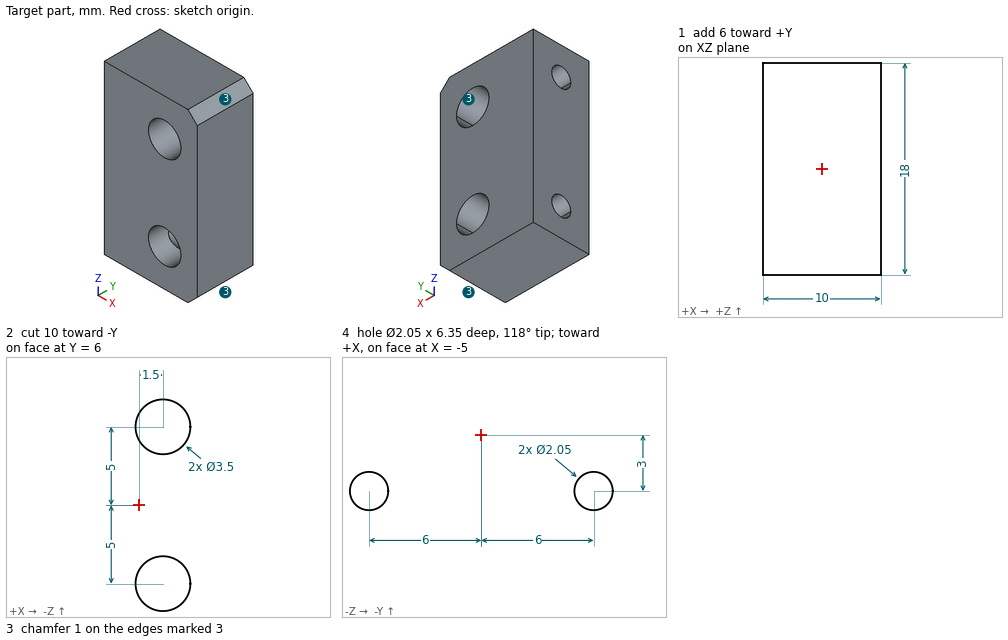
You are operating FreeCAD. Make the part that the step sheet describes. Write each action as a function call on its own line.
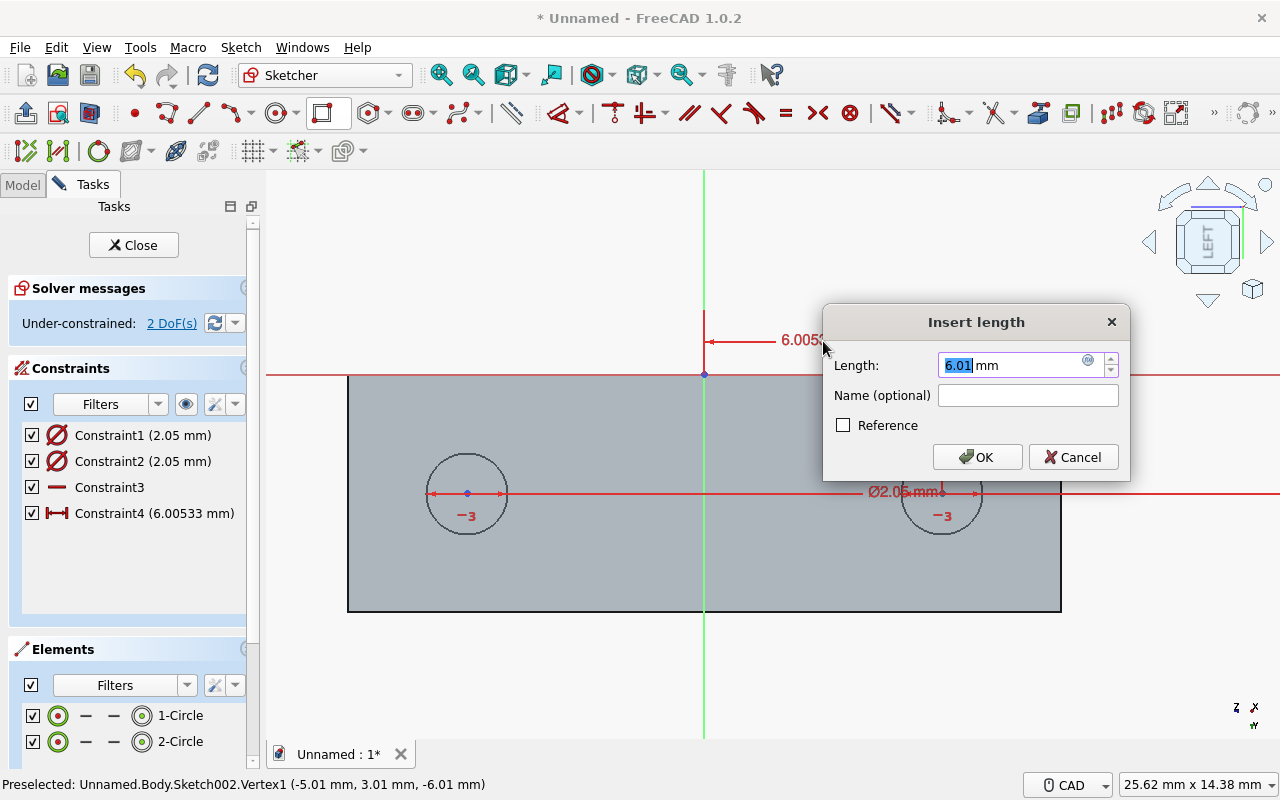
text(6)
key(Return)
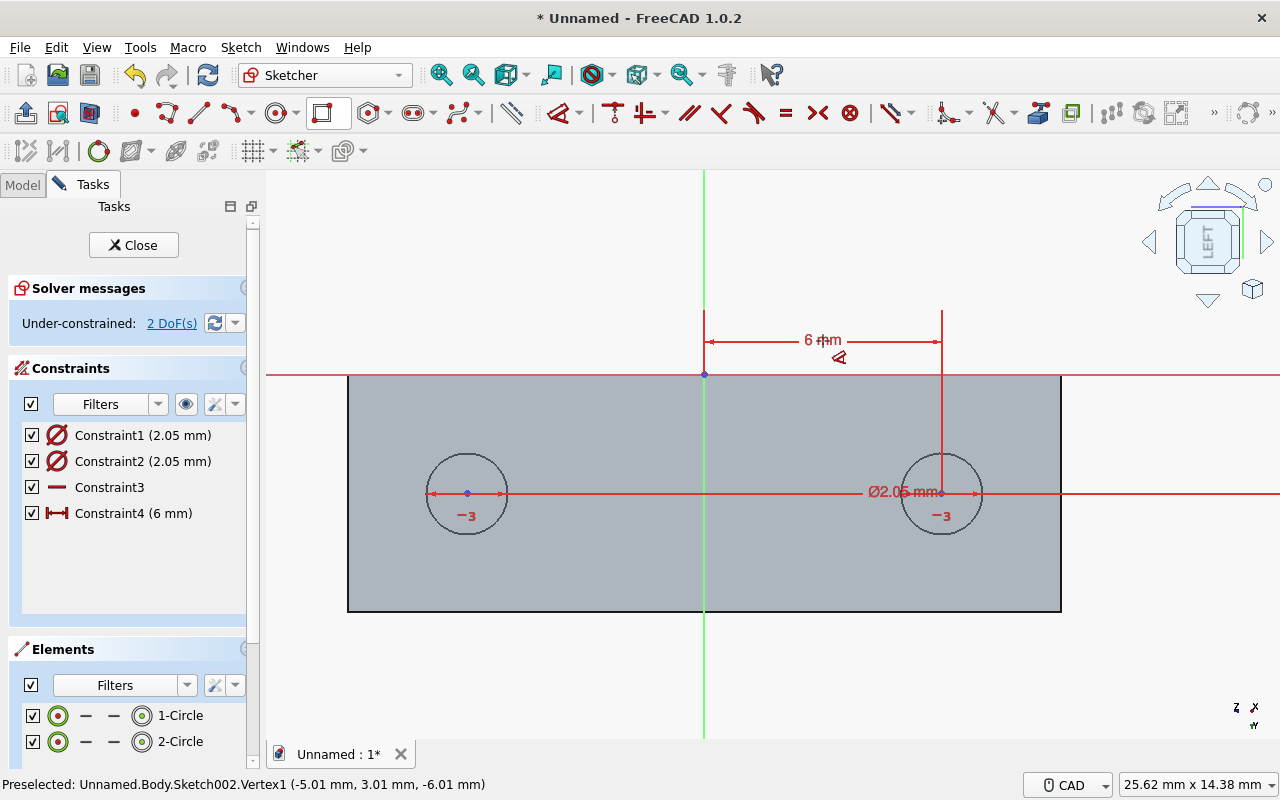
click(942, 494)
click(976, 434)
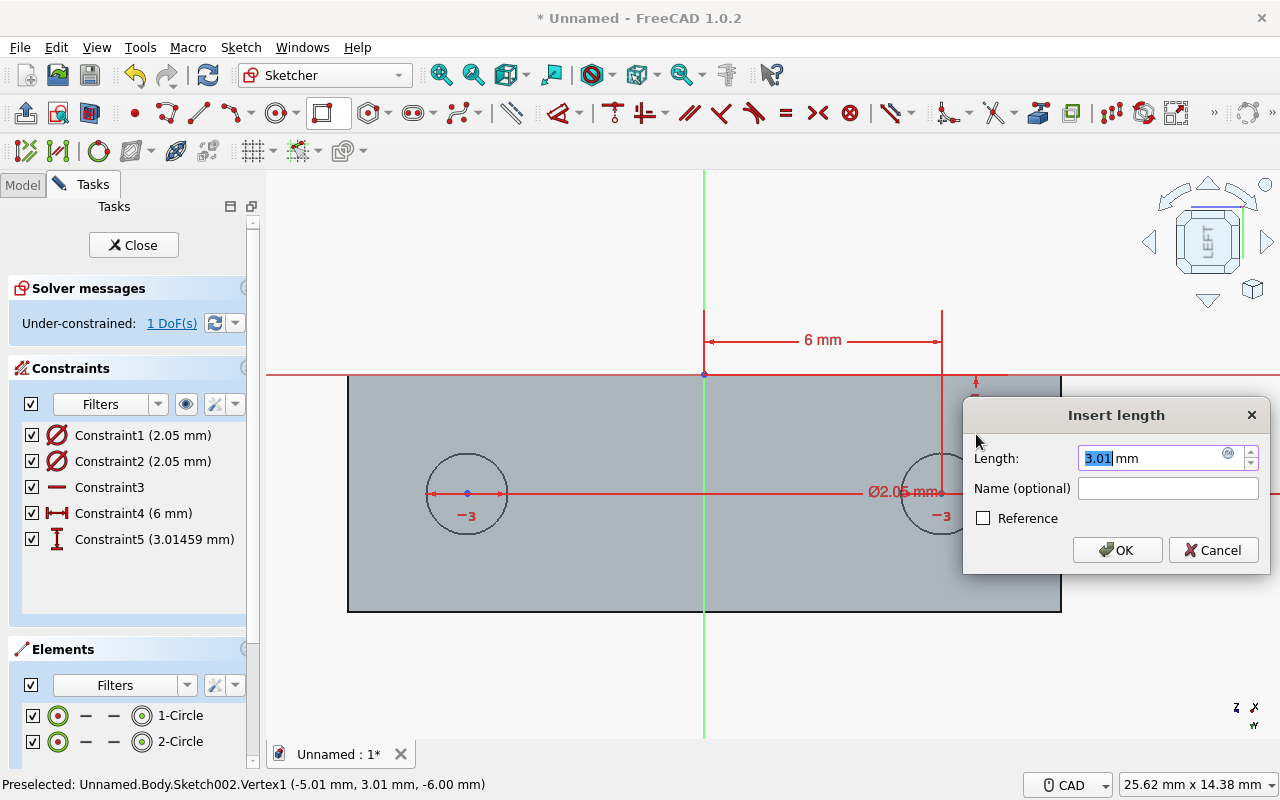
text(3)
key(Return)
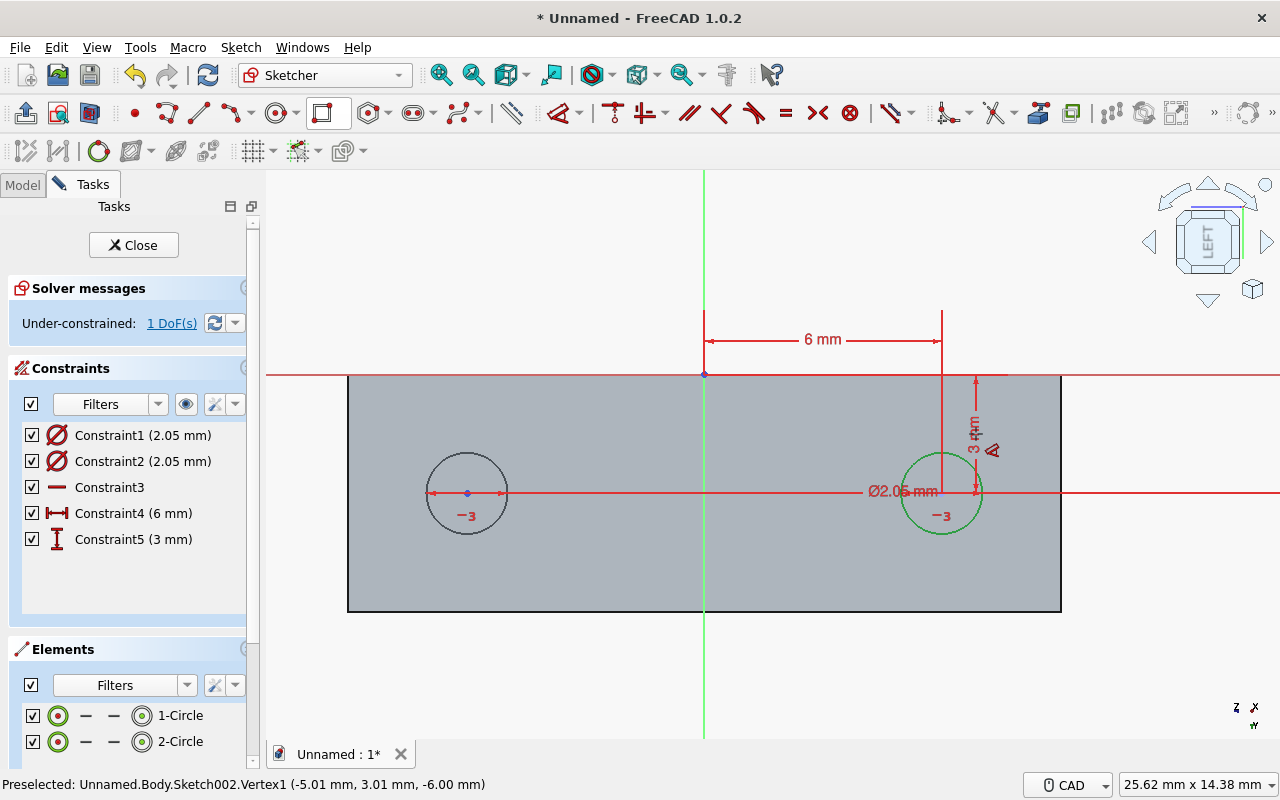
click(467, 493)
click(586, 341)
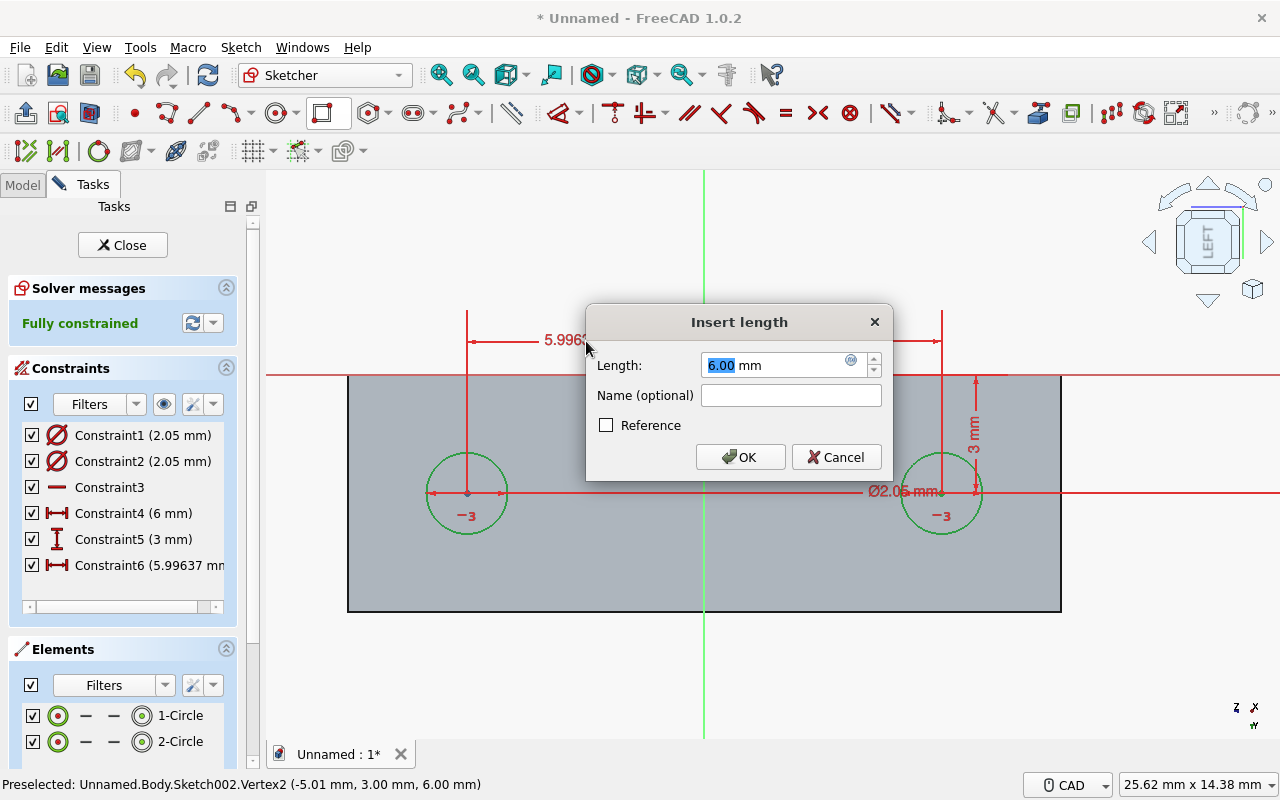
text(6)
key(Return)
key(Escape)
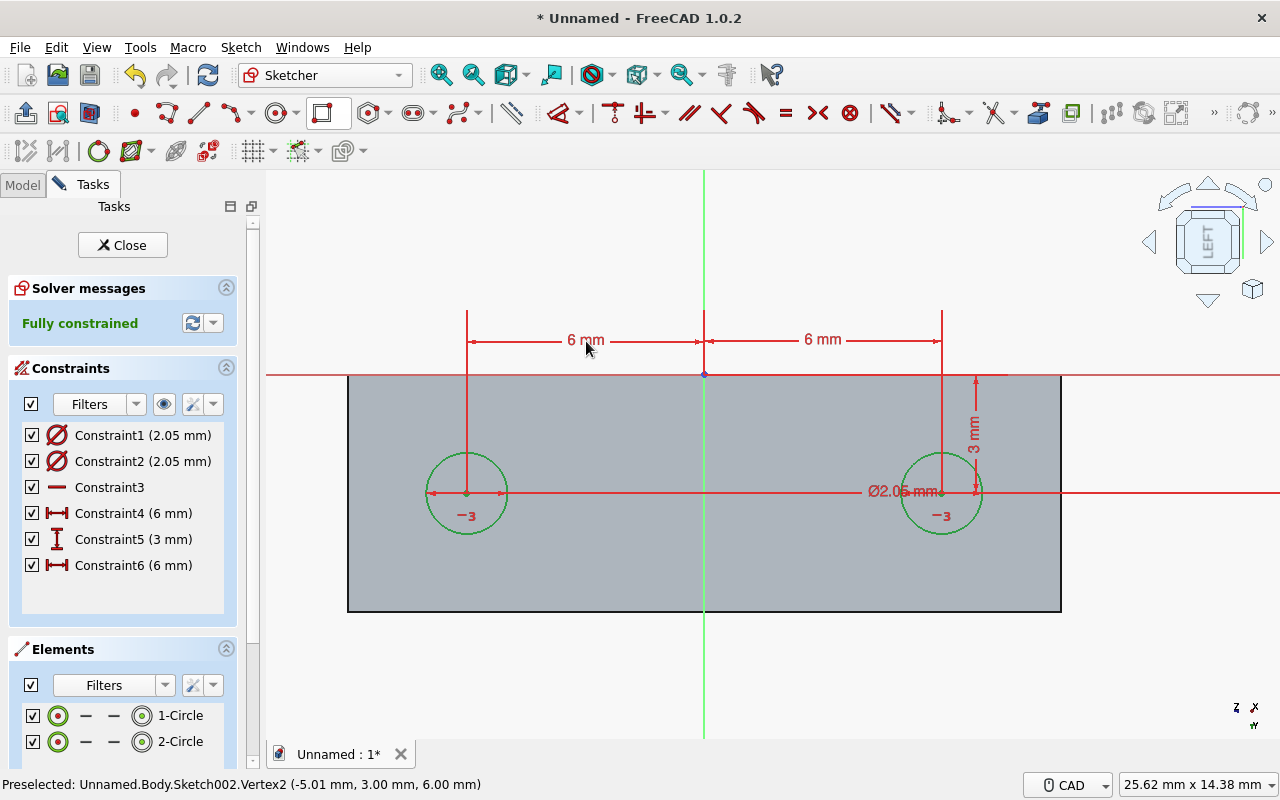
click(123, 245)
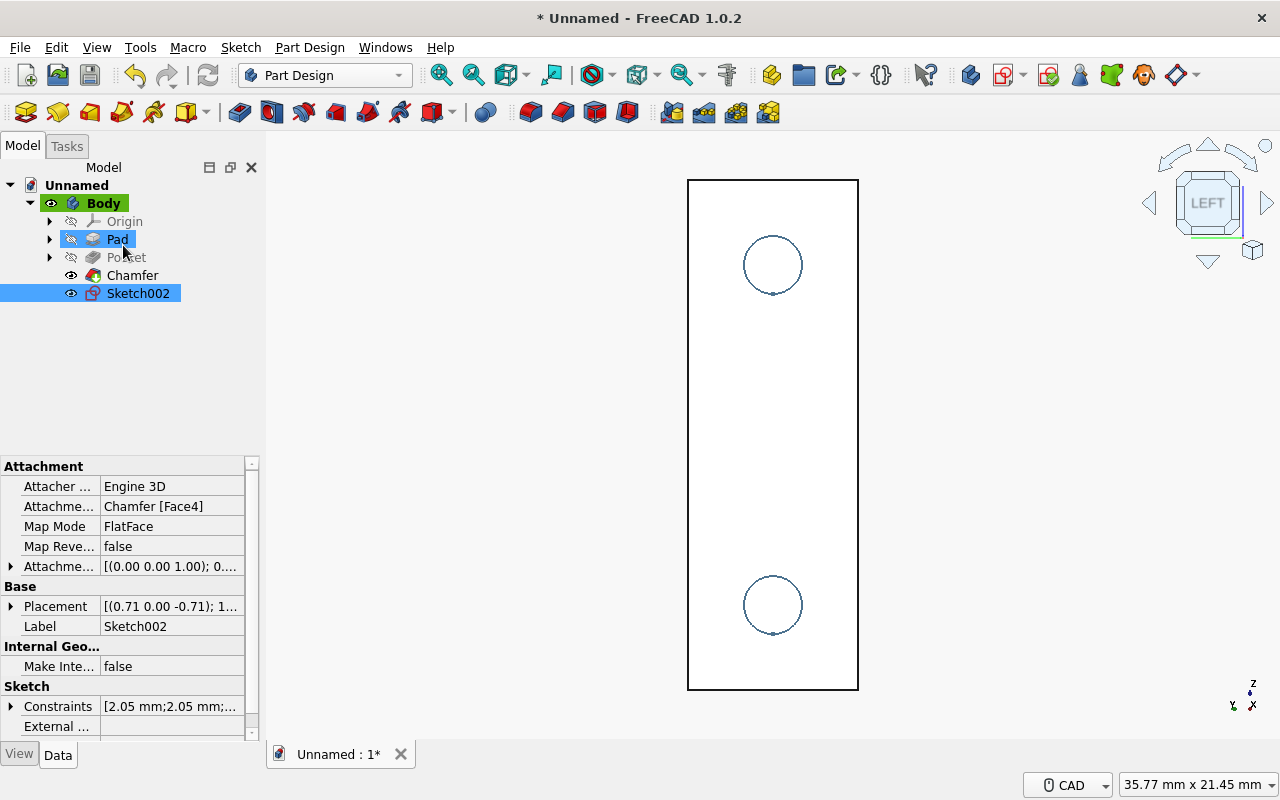
click(272, 112)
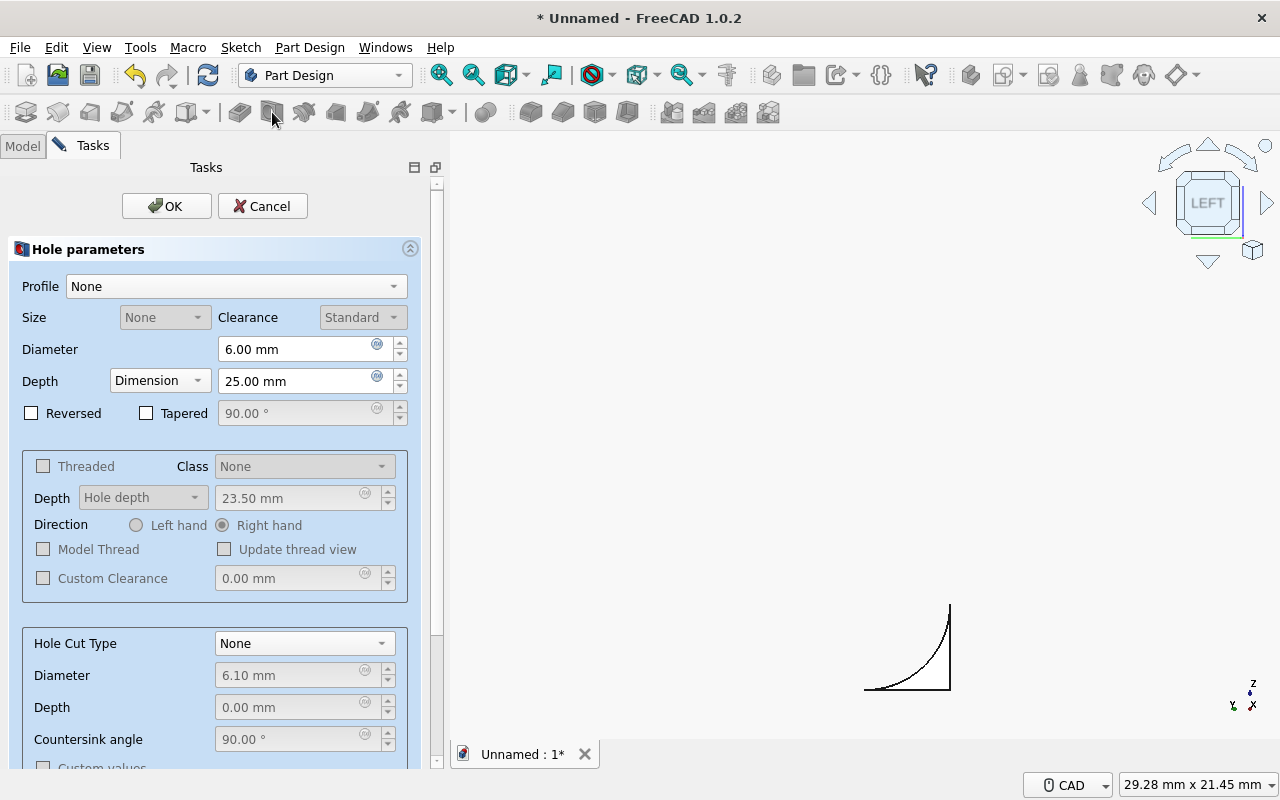
triple_click(305, 349)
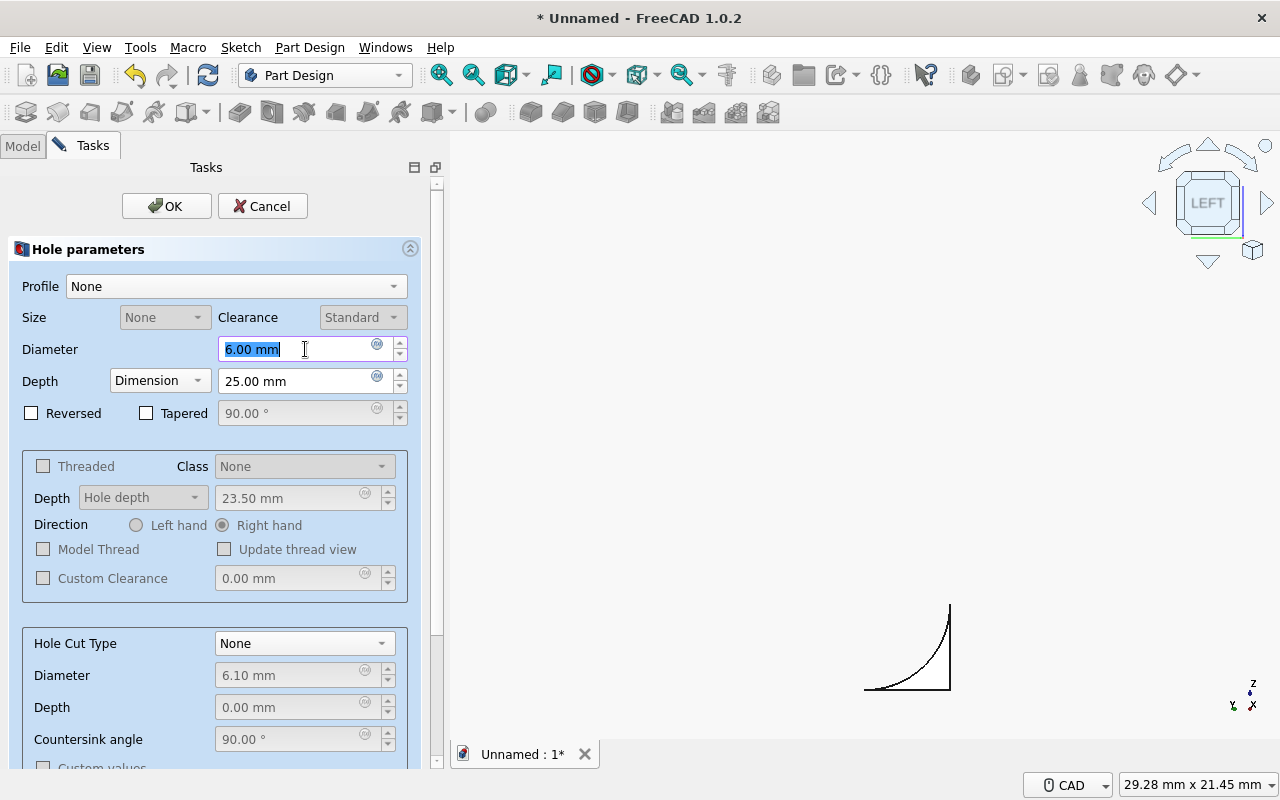
text(2.05)
key(Tab)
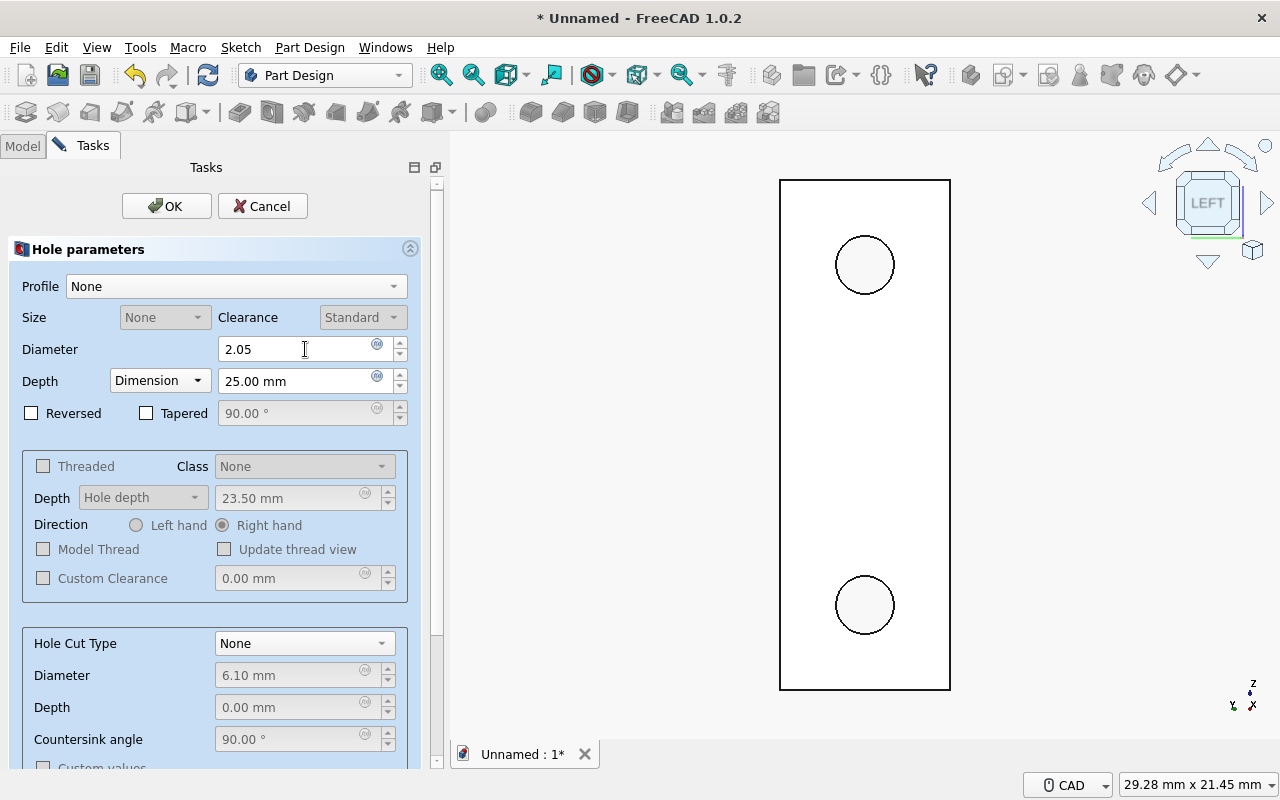
triple_click(305, 381)